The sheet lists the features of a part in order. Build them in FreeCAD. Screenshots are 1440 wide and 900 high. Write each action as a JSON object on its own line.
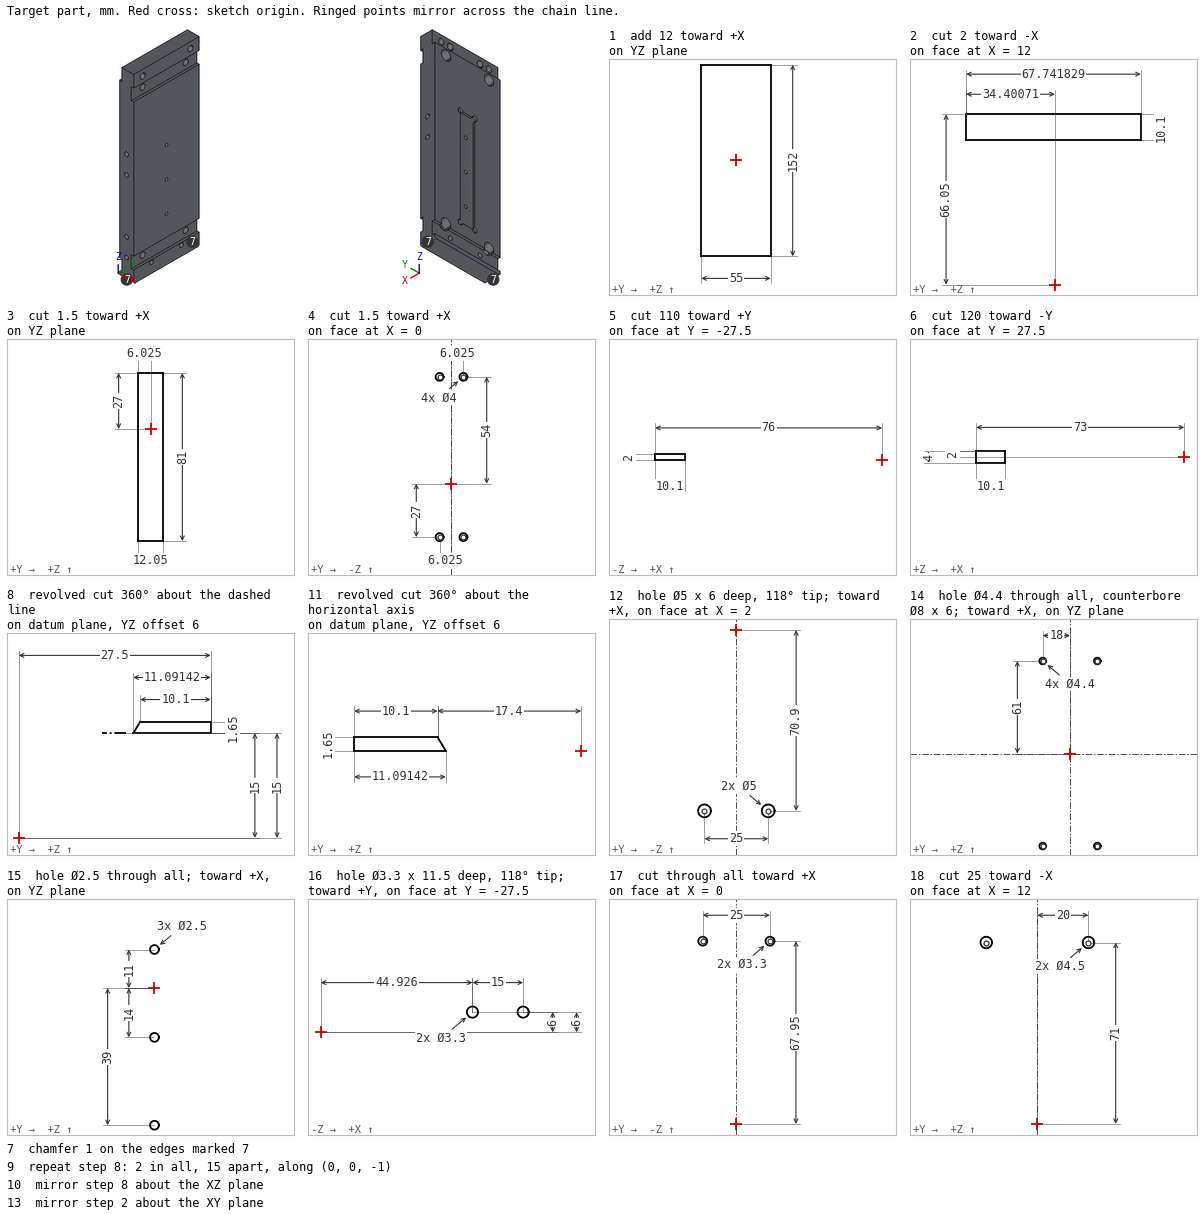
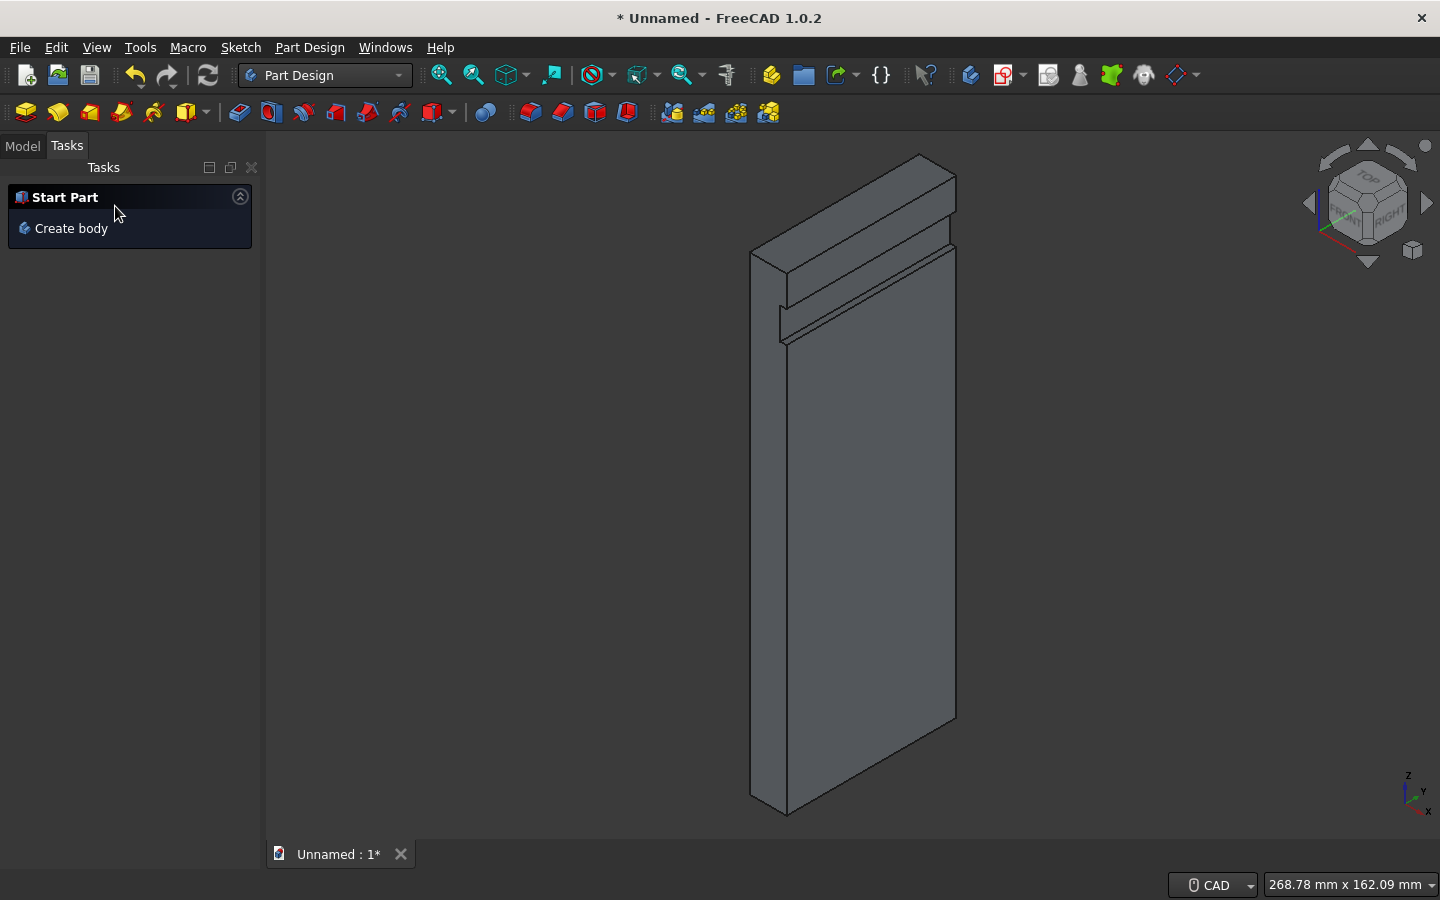
{"action": "left_click", "coordinate": [768, 765]}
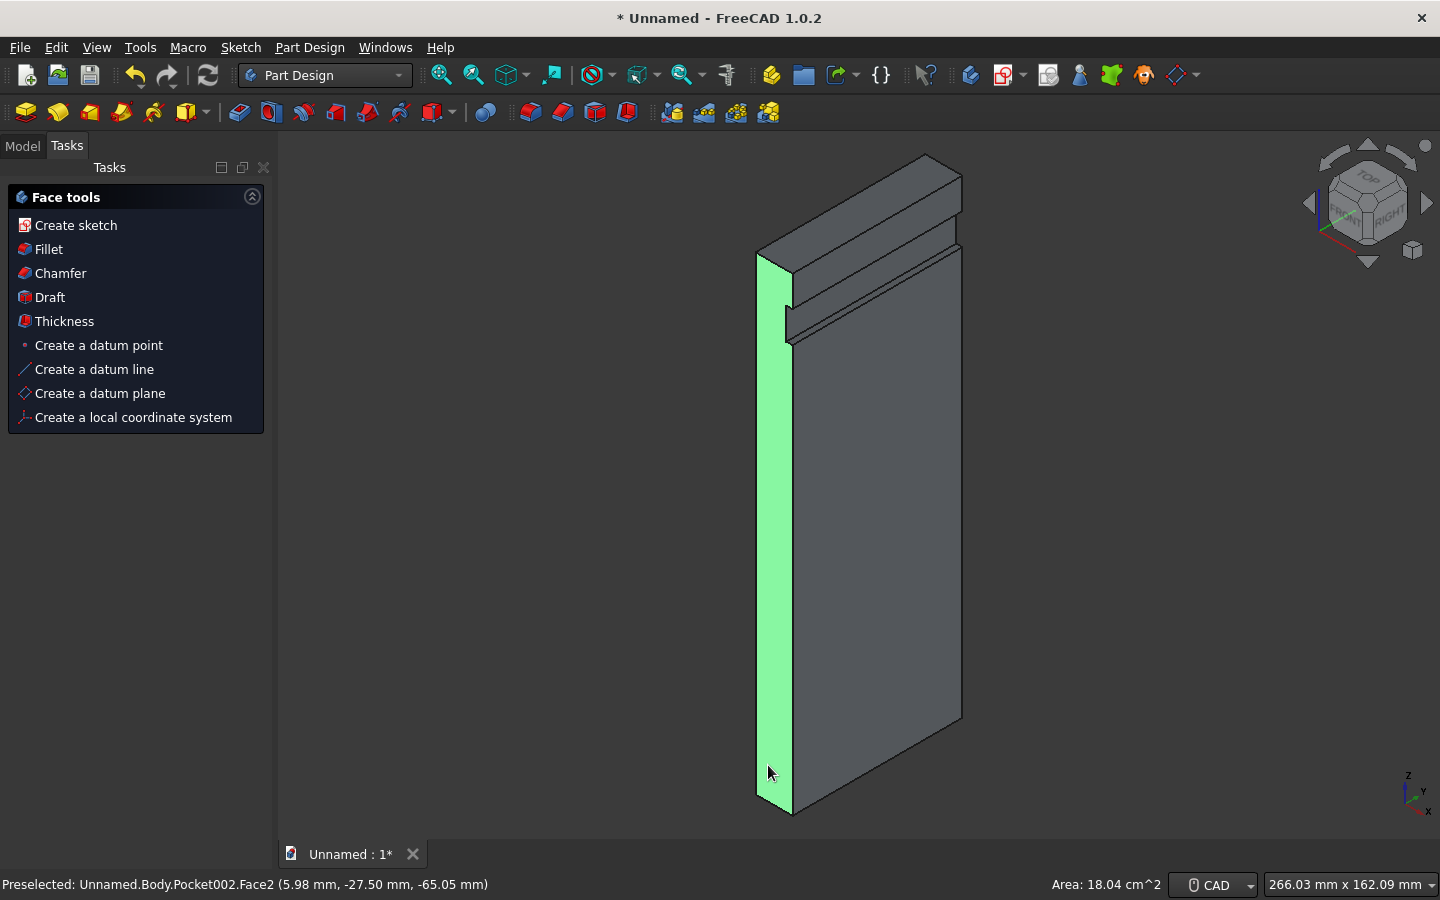
{"action": "left_click", "coordinate": [1004, 76]}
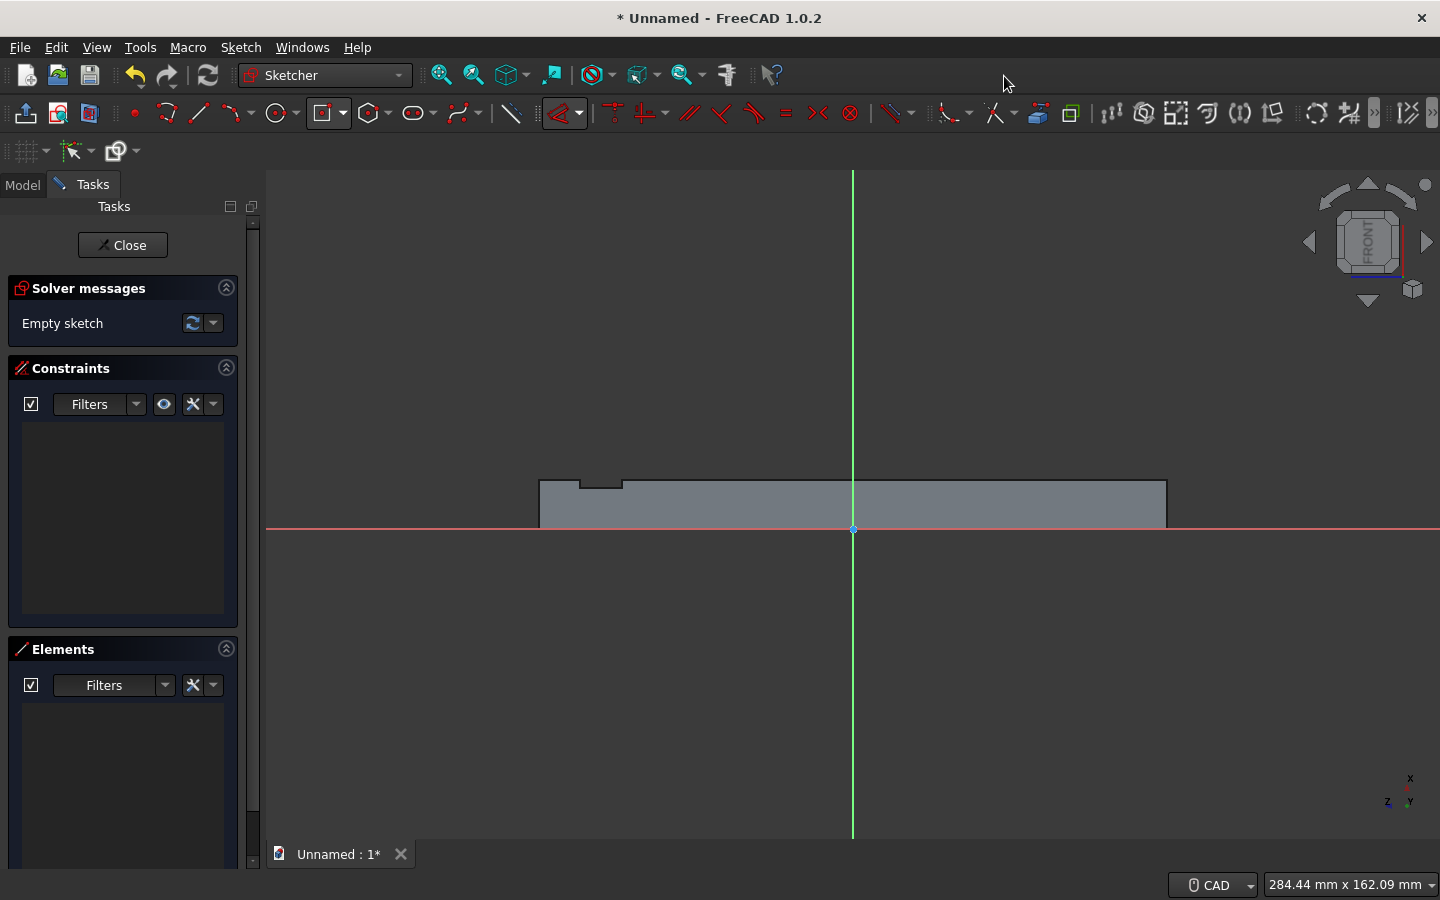
{"action": "scroll", "coordinate": [546, 526], "scroll_direction": "up", "scroll_amount": 14}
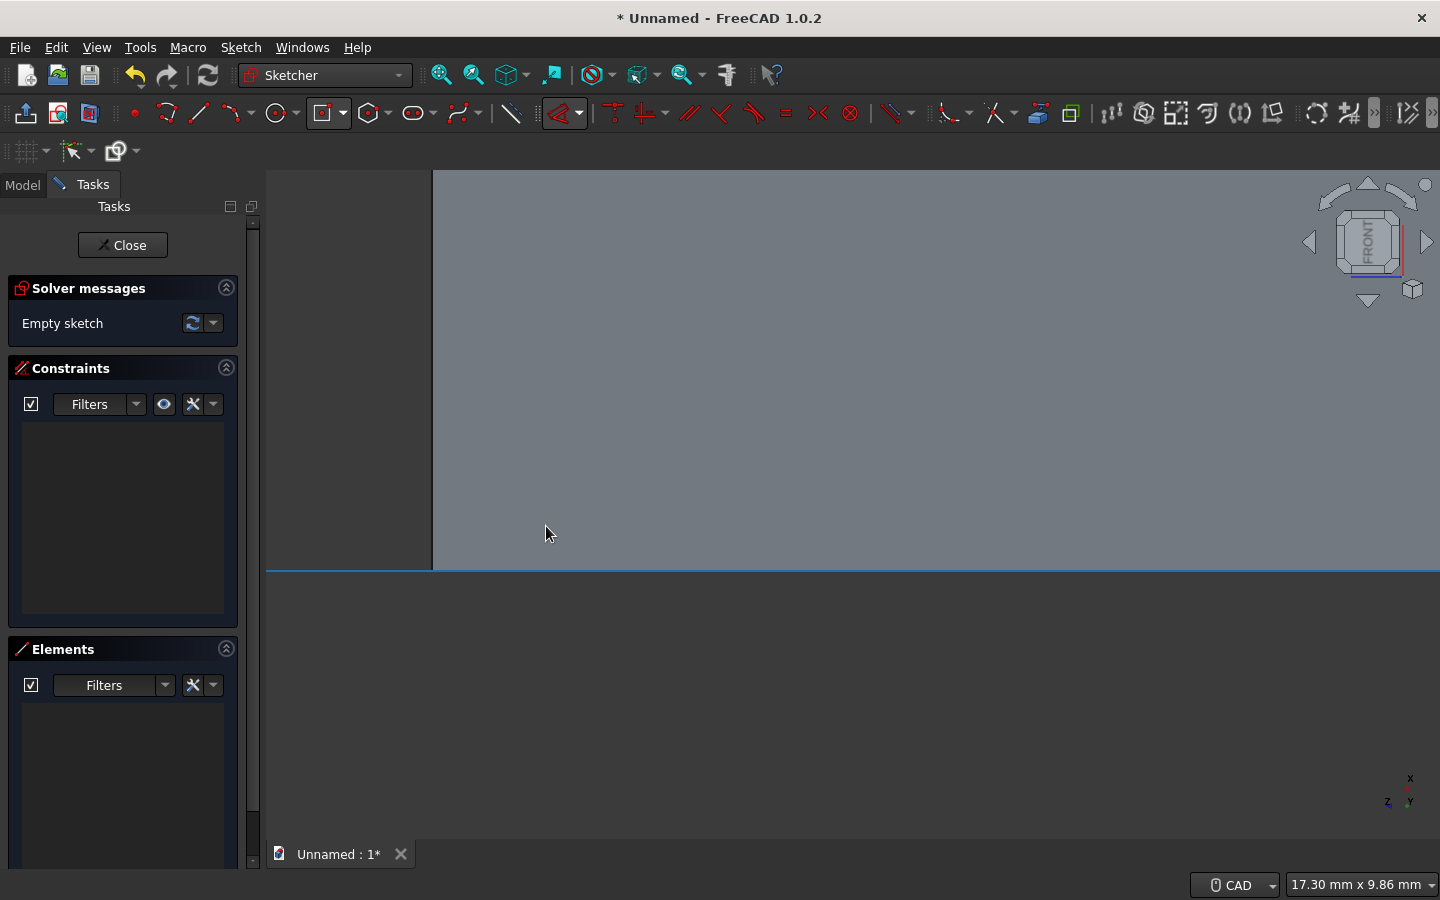
{"action": "key", "text": "g r"}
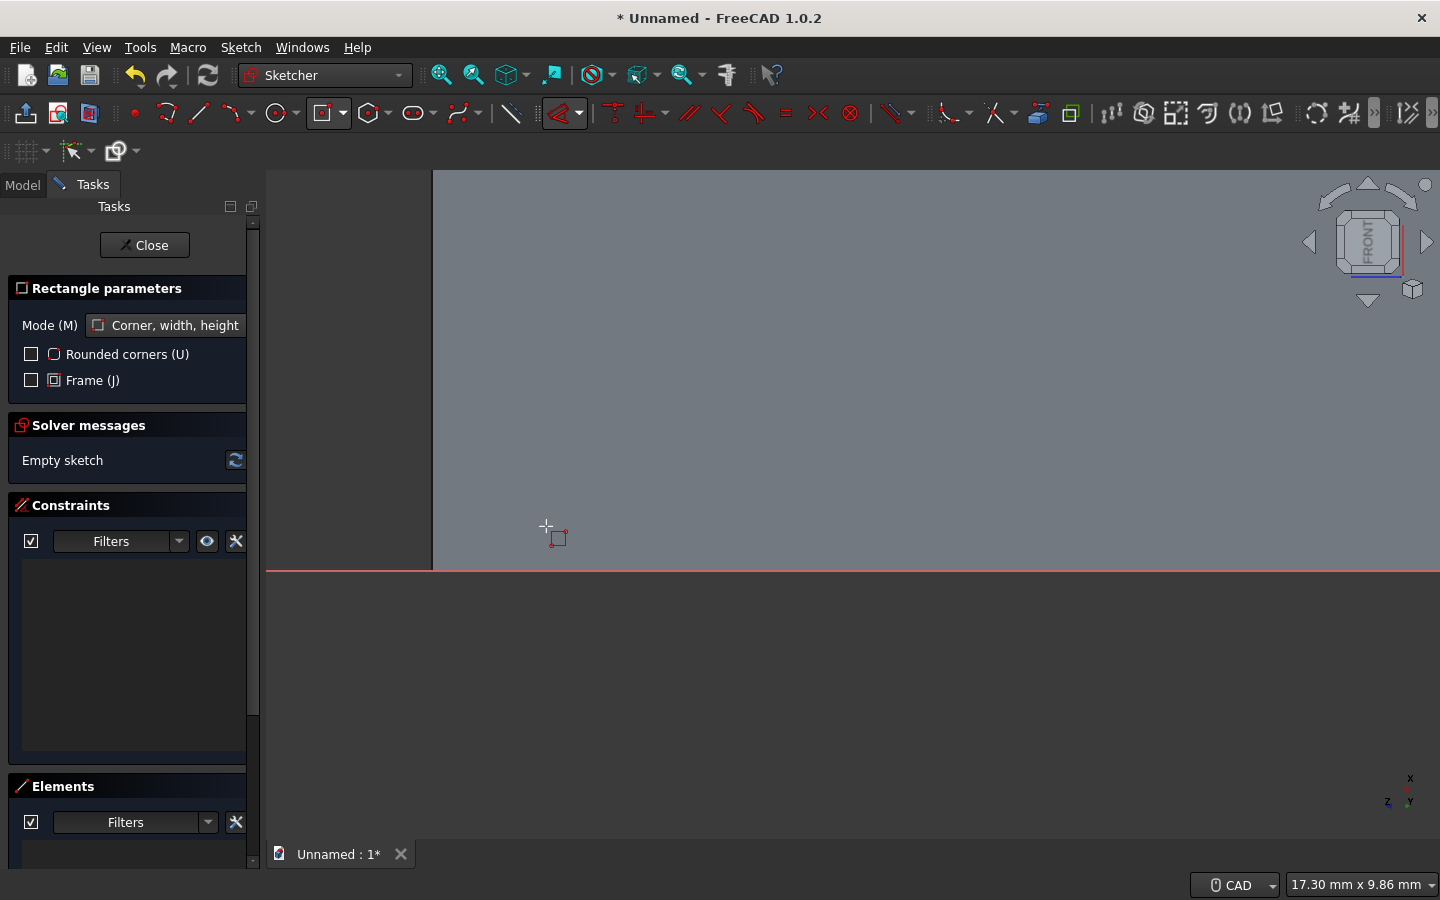
{"action": "left_click", "coordinate": [432, 436]}
{"action": "left_click", "coordinate": [1118, 571]}
{"action": "key", "text": "Escape"}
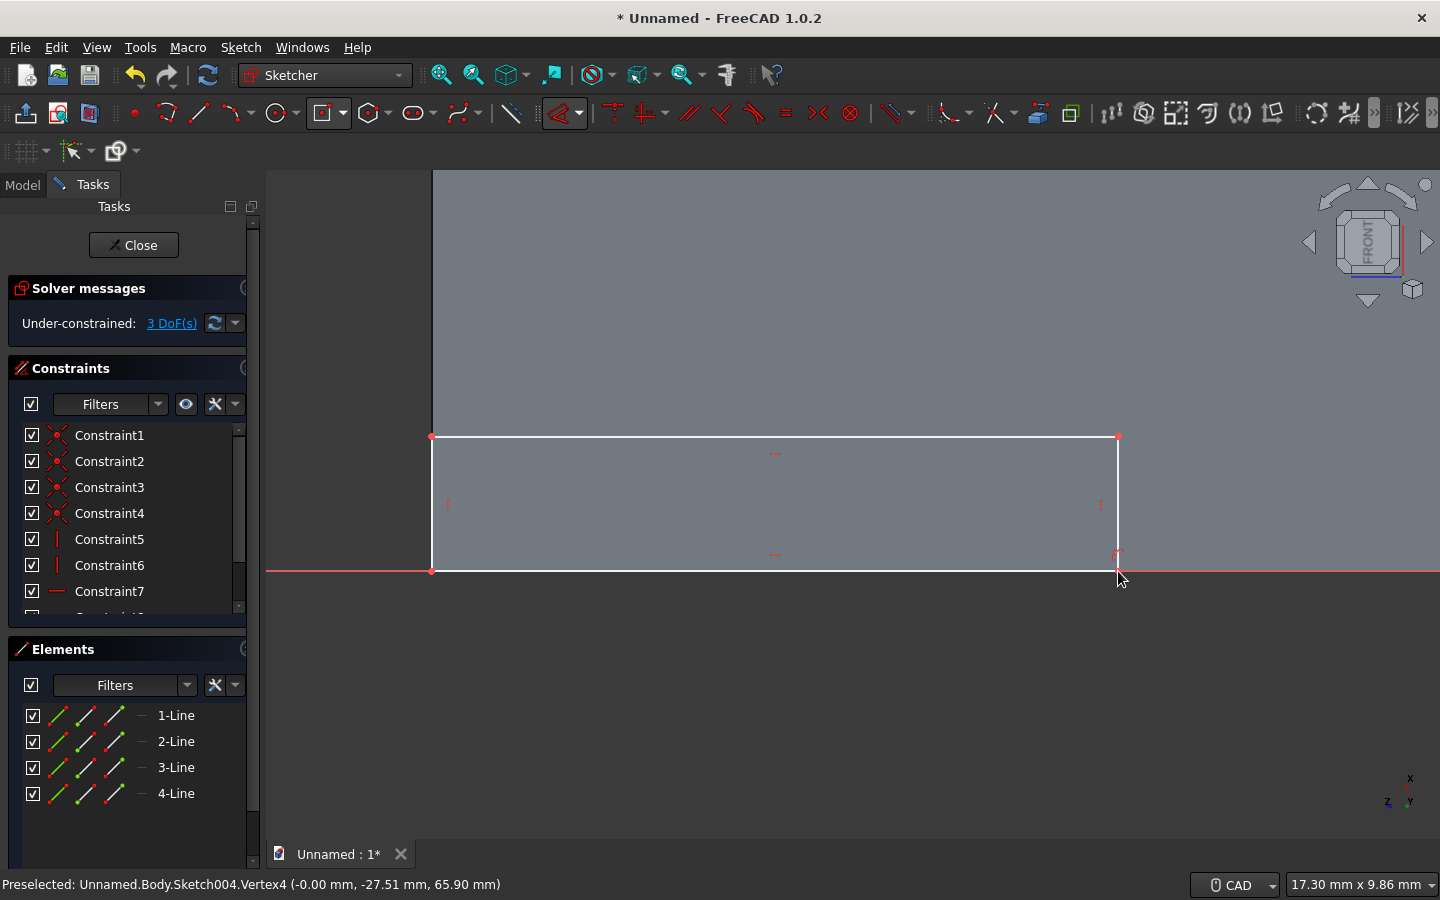
{"action": "left_click", "coordinate": [432, 477]}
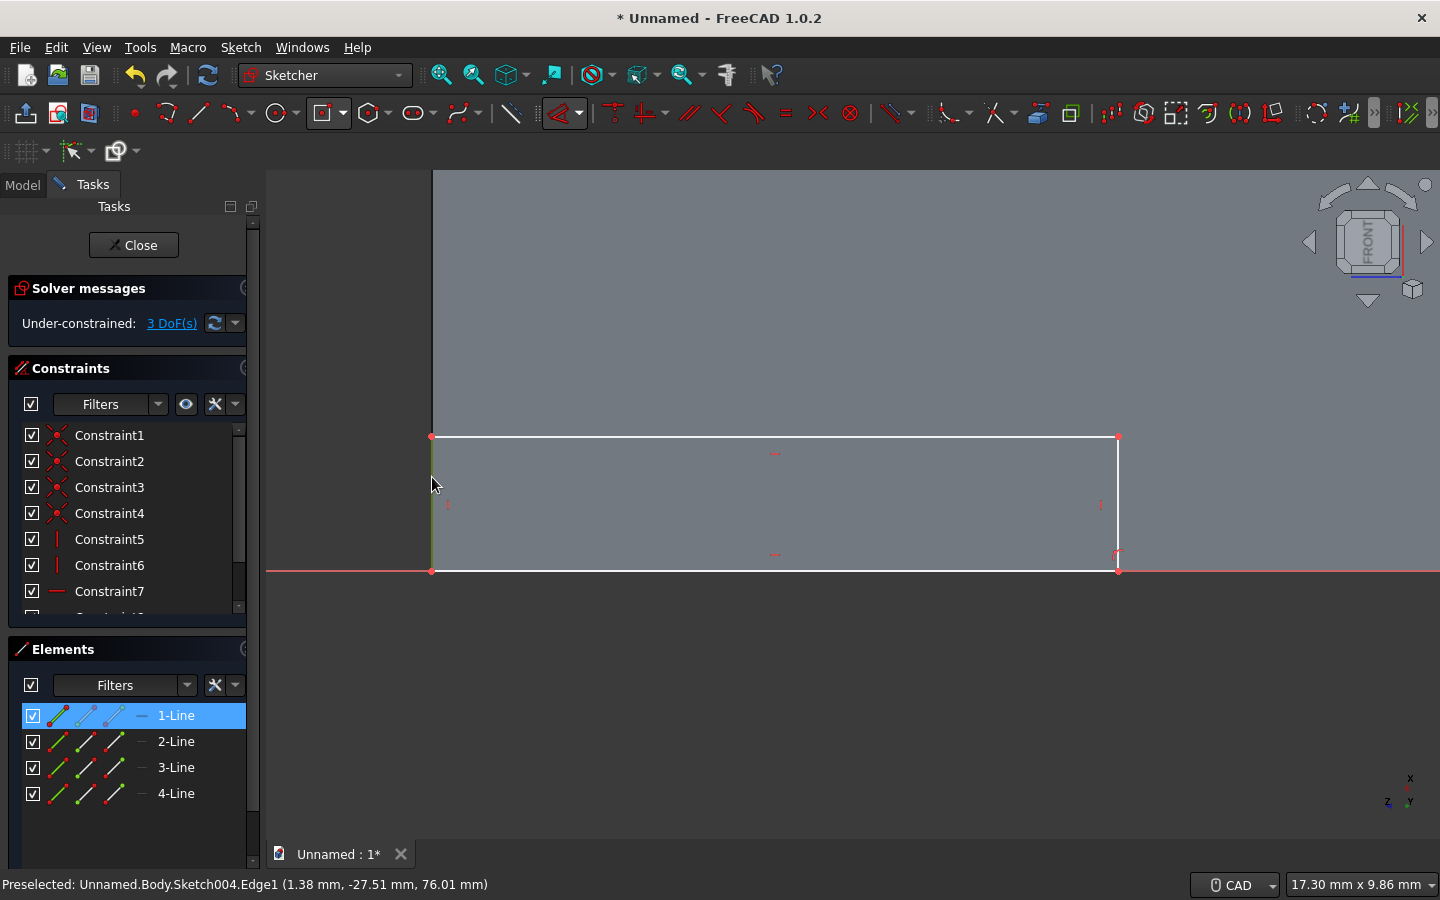
{"action": "key", "text": "i"}